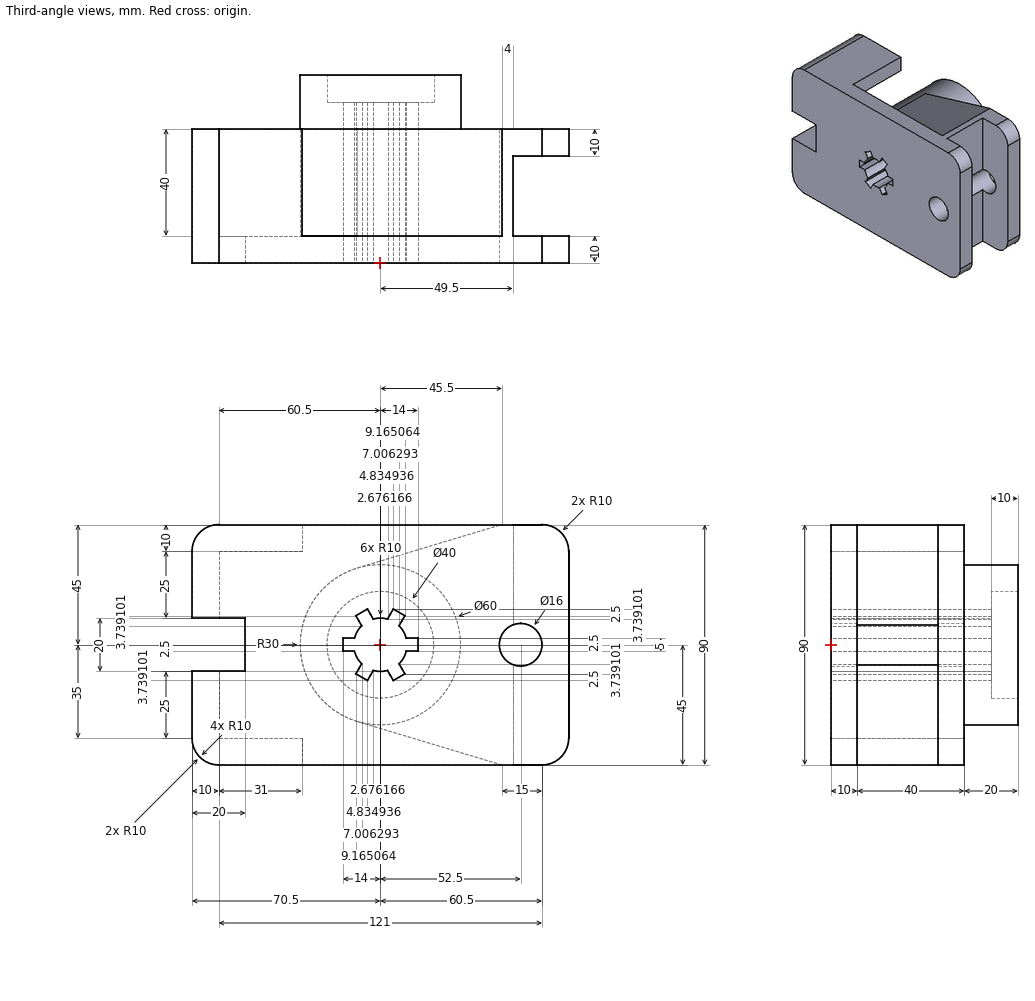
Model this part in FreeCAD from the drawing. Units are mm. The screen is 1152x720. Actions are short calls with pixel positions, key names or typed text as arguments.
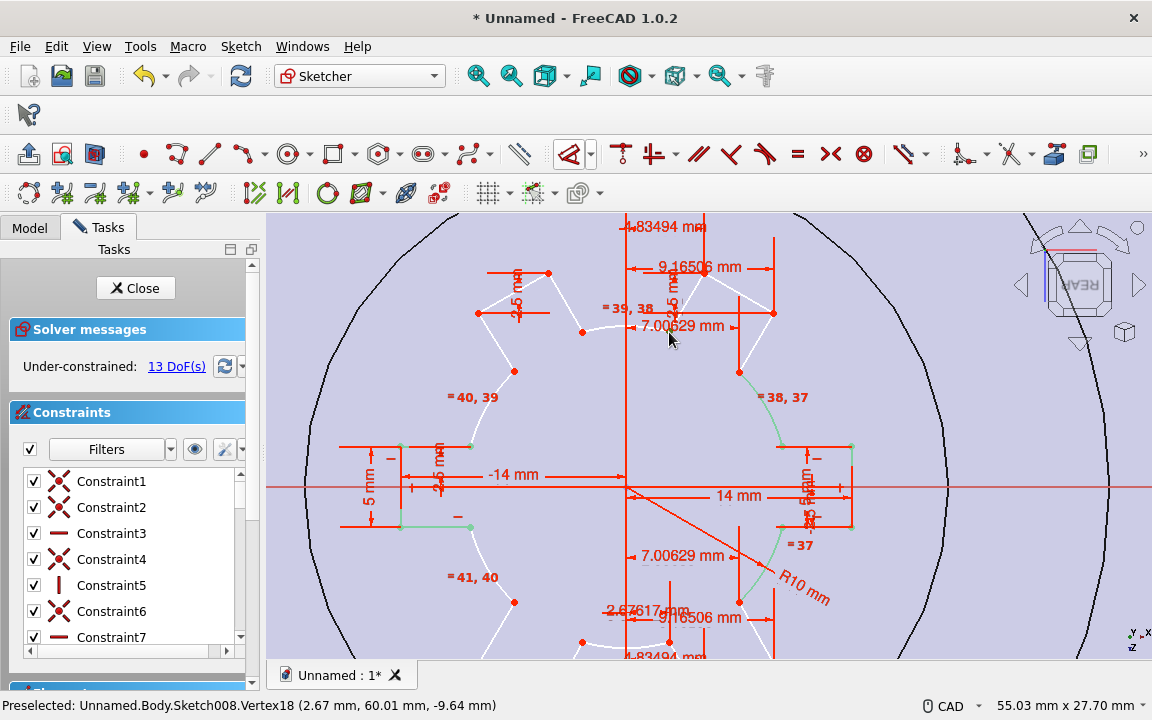
click(590, 154)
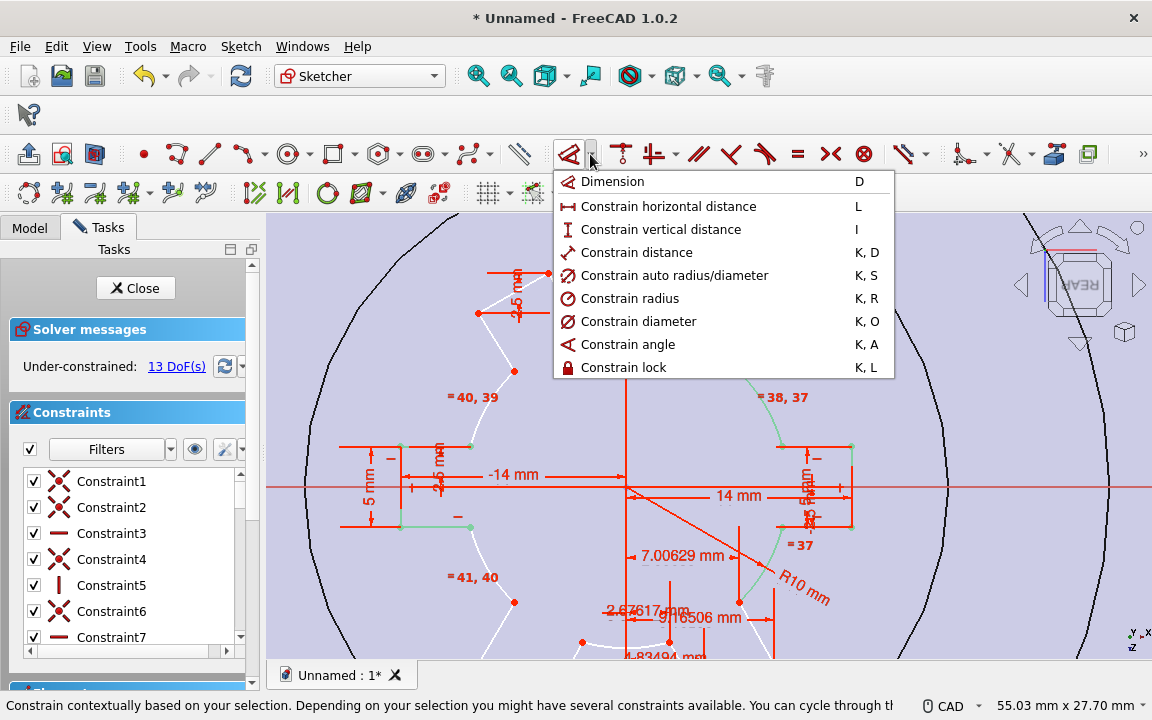
click(724, 206)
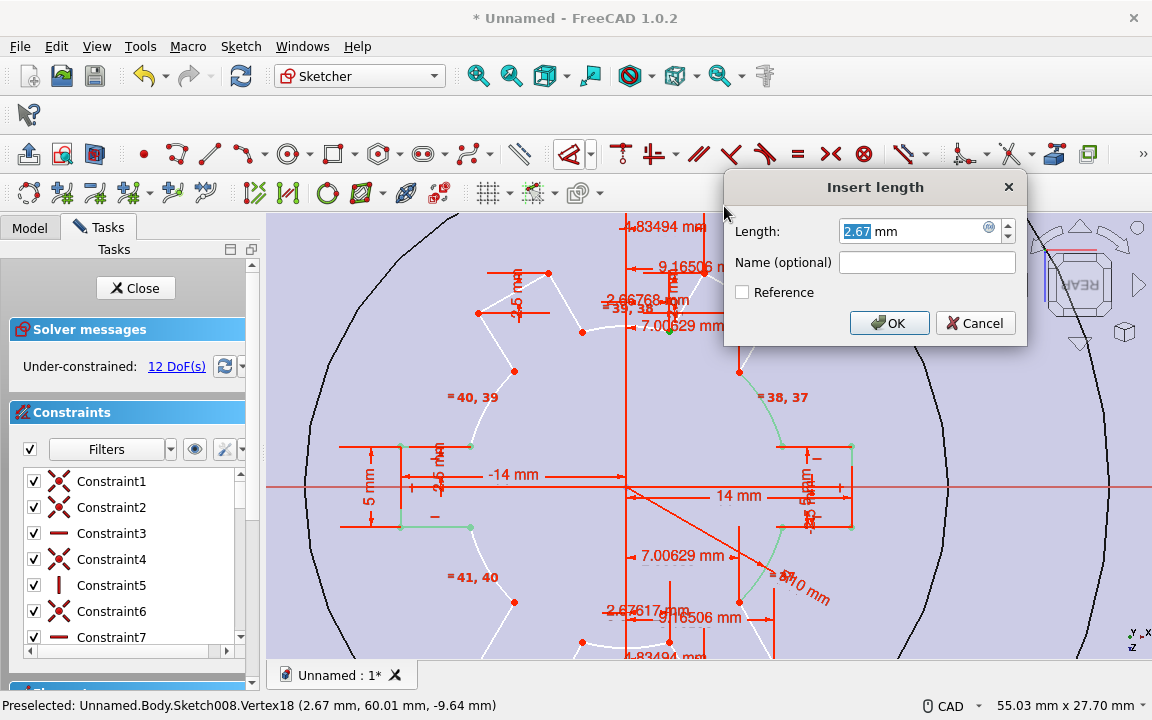
text(2.676166)
key(Return)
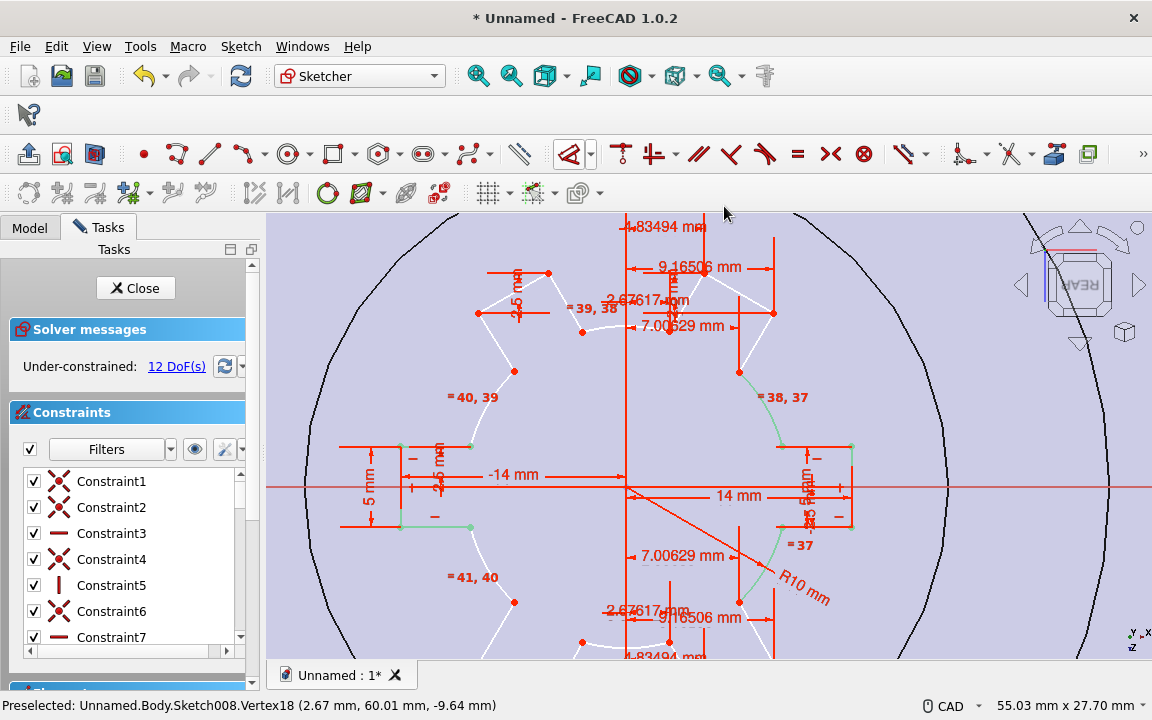
click(583, 332)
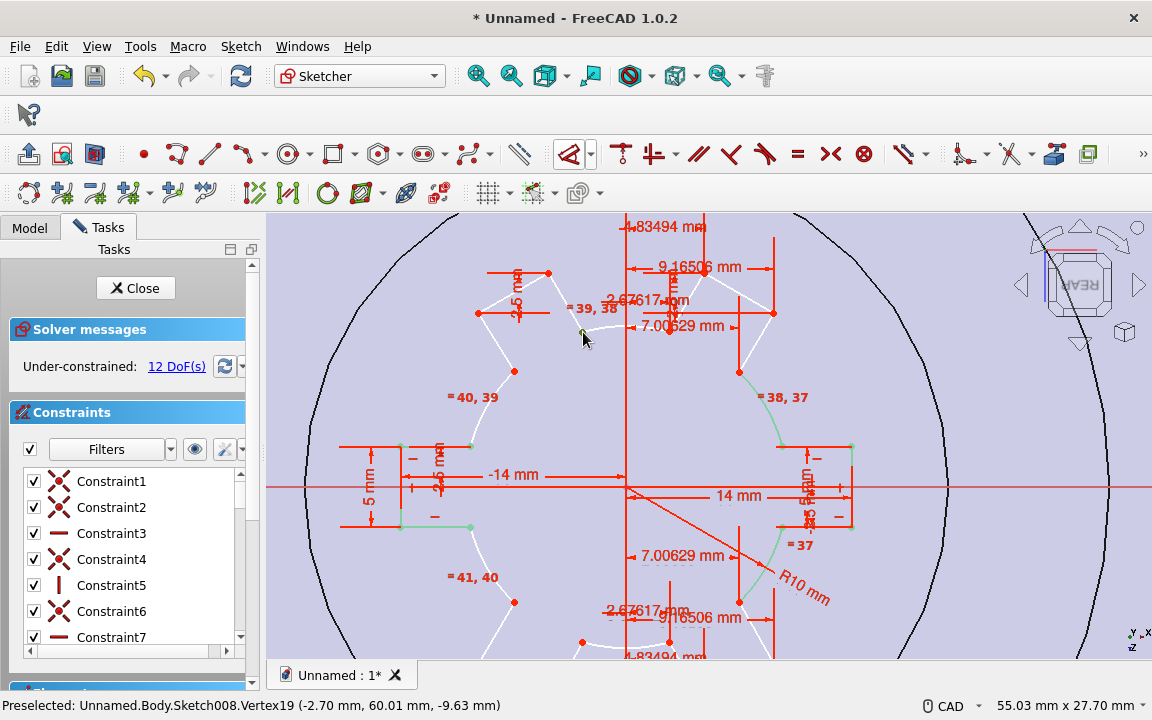
key(l)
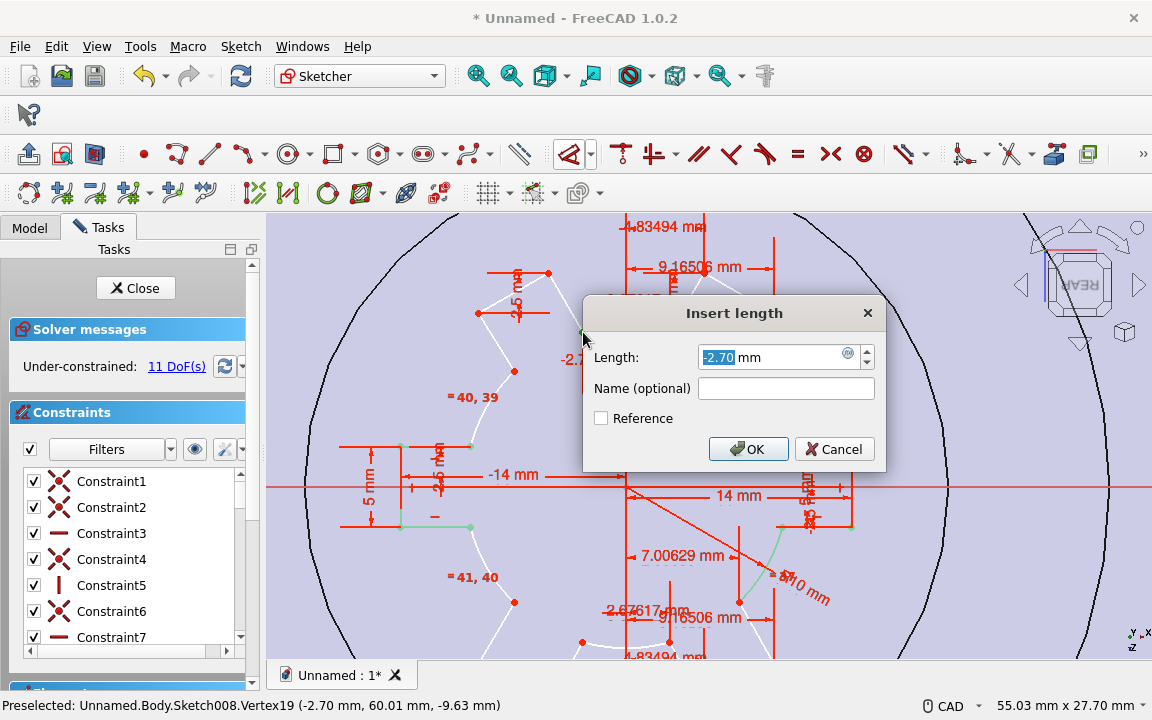
text(-2.676166)
key(Return)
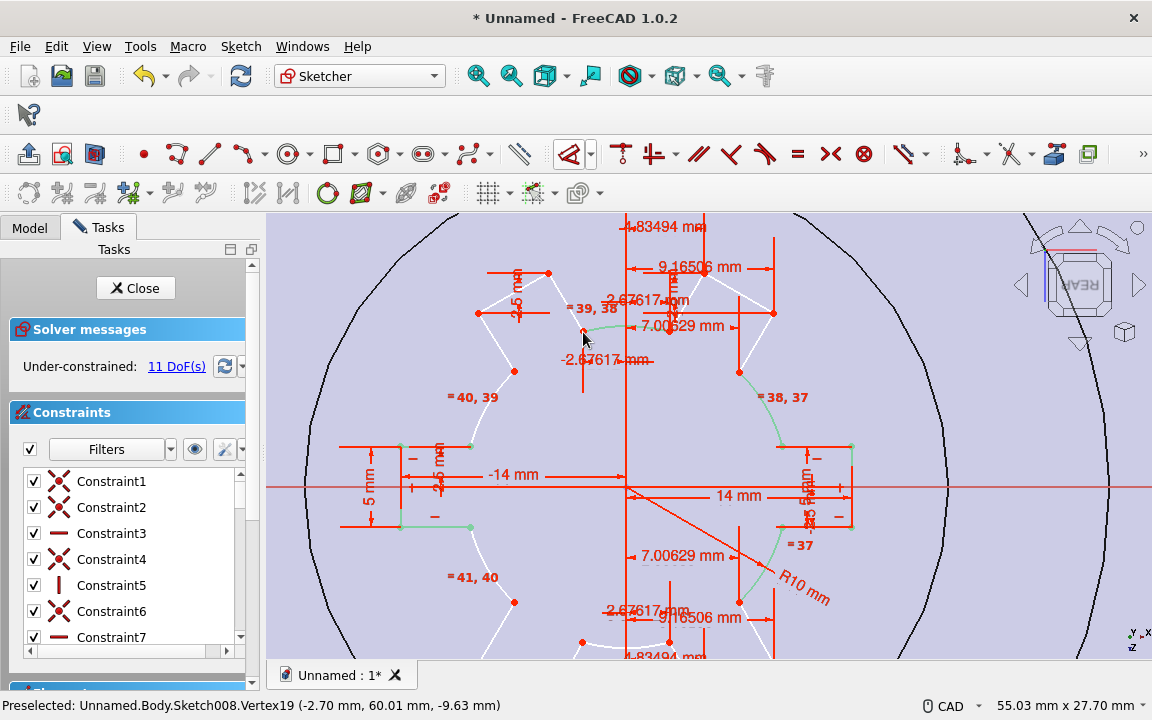
click(549, 273)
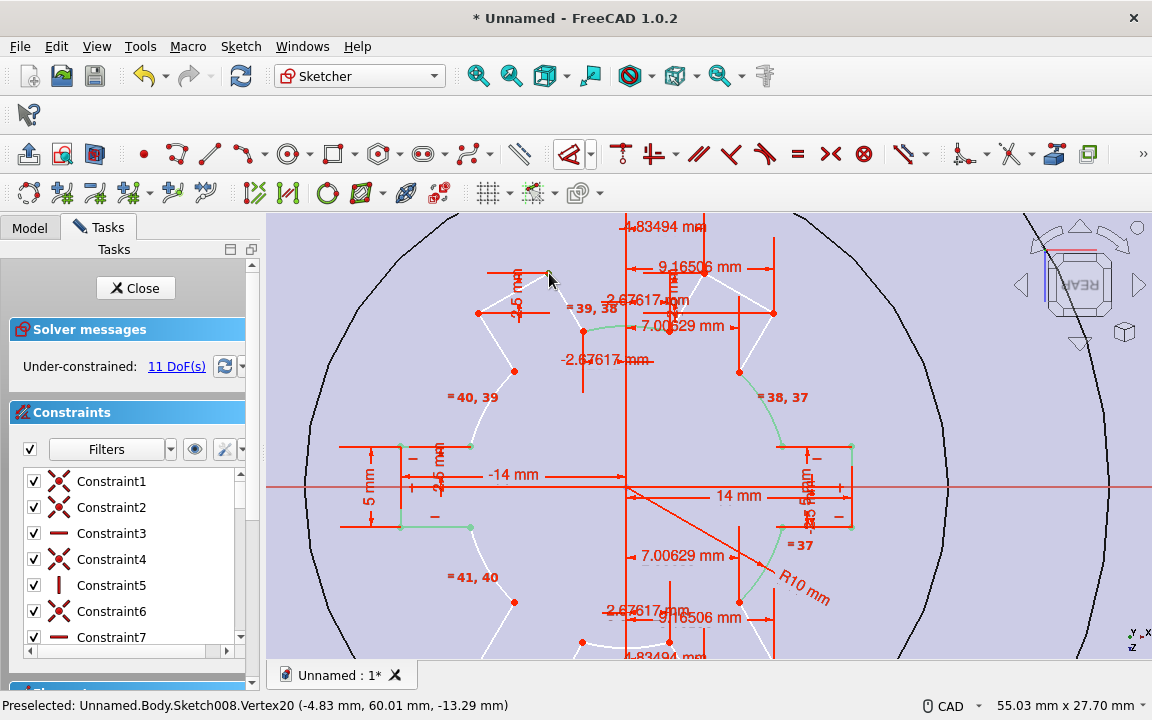
click(590, 154)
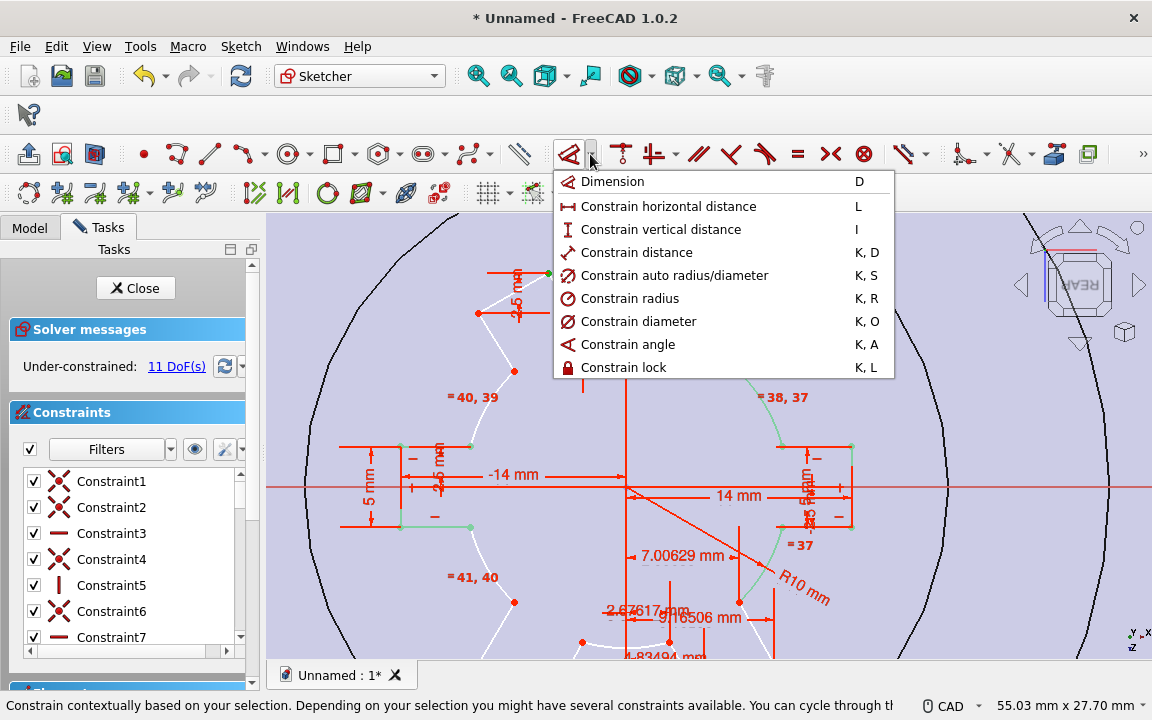
click(724, 206)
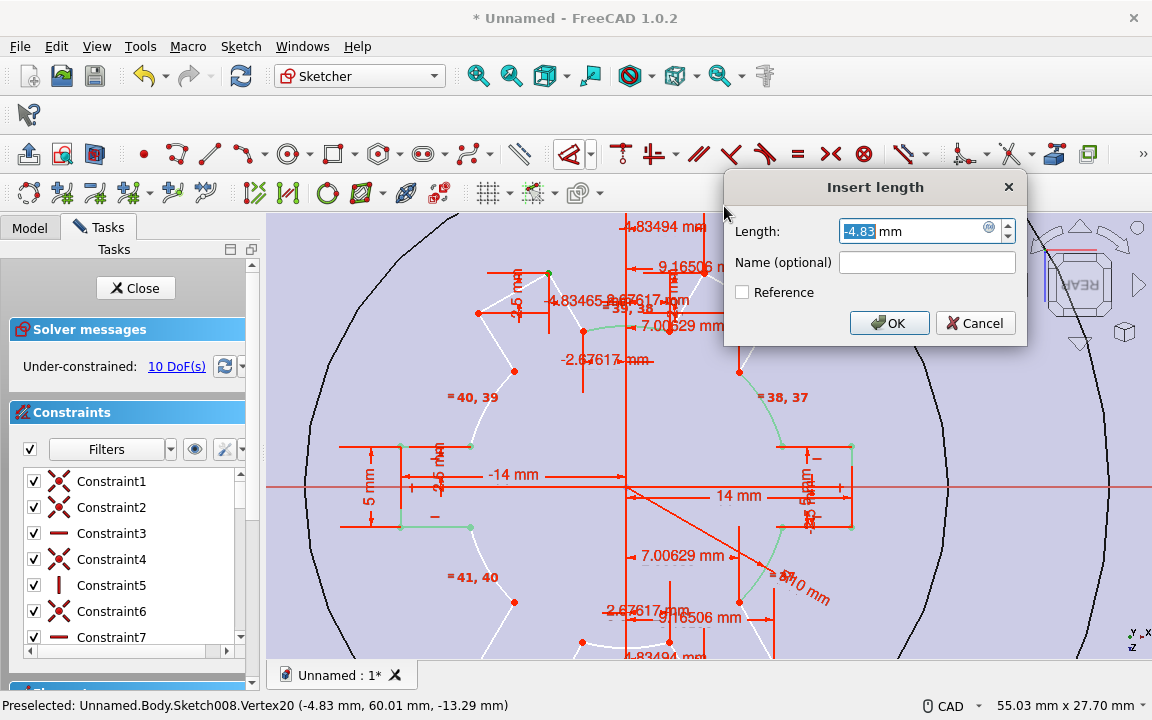
text(-4.834936)
key(Return)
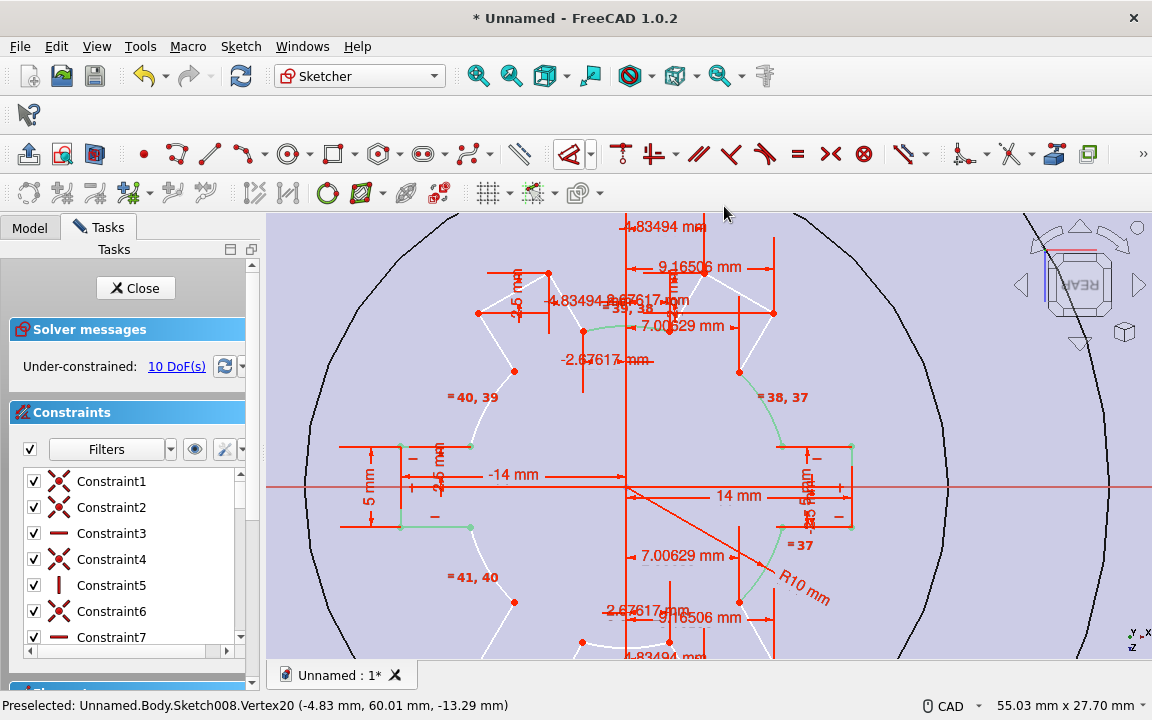
click(478, 313)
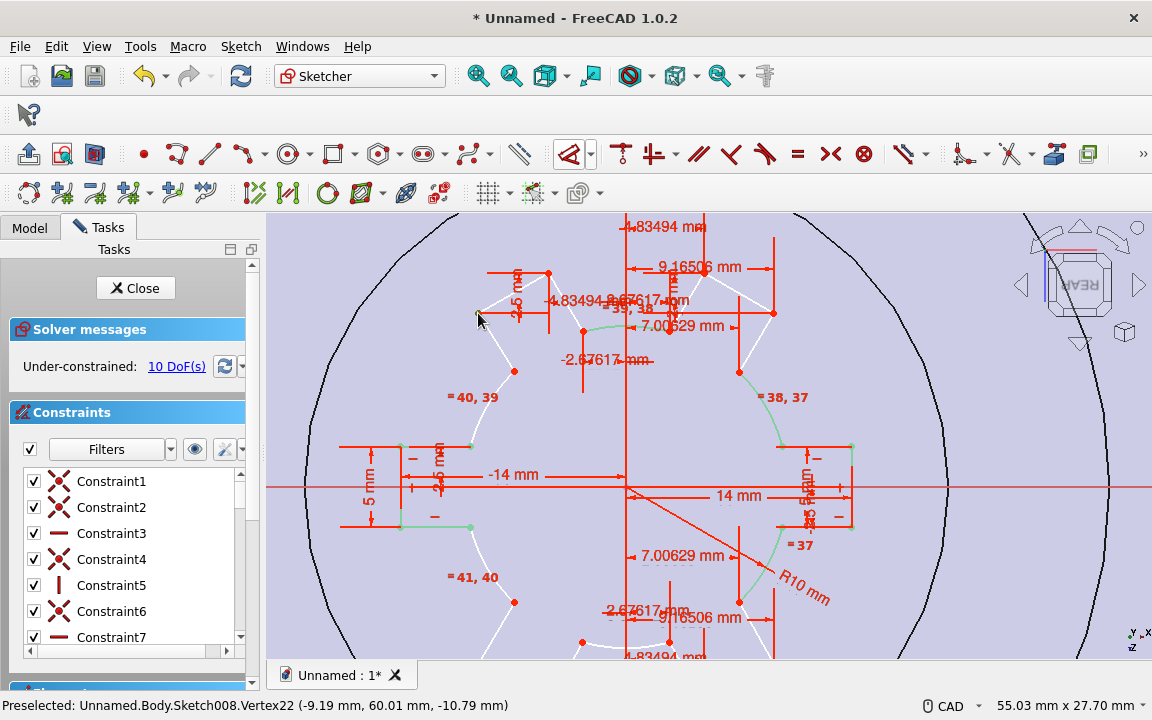
click(590, 154)